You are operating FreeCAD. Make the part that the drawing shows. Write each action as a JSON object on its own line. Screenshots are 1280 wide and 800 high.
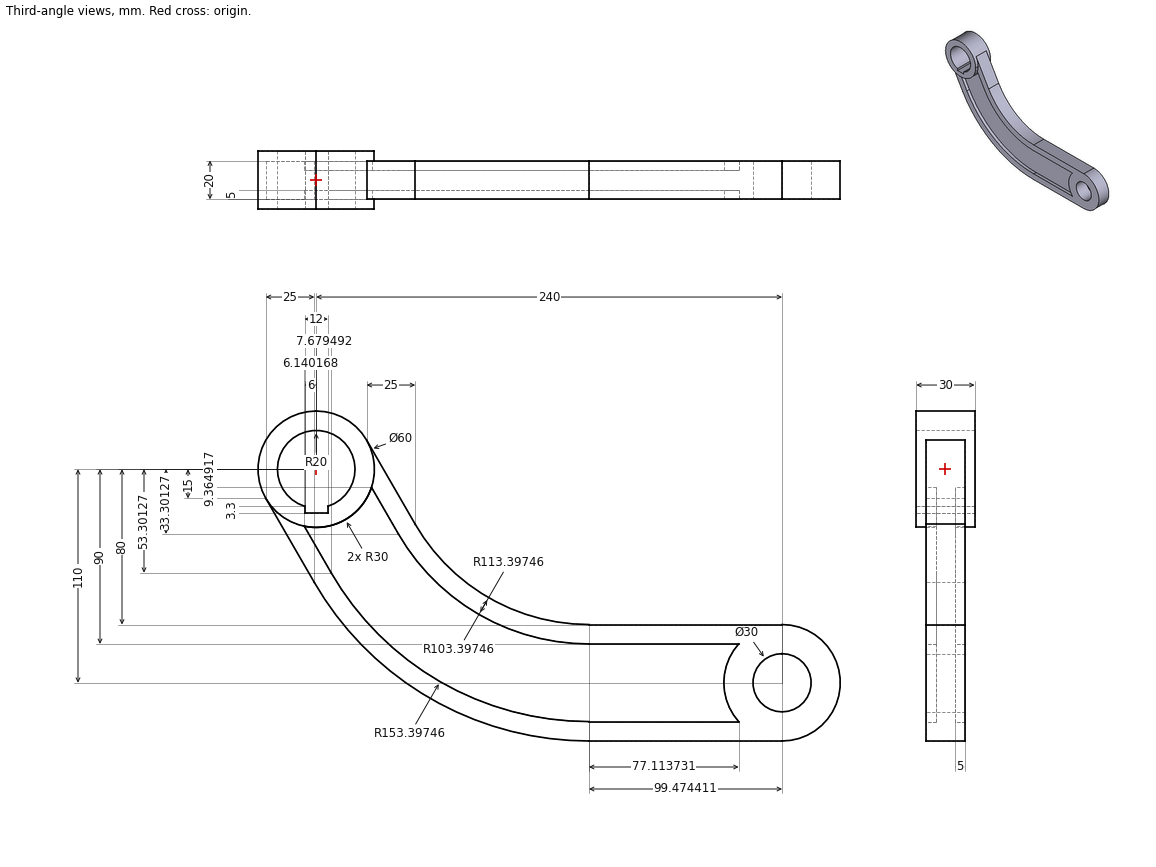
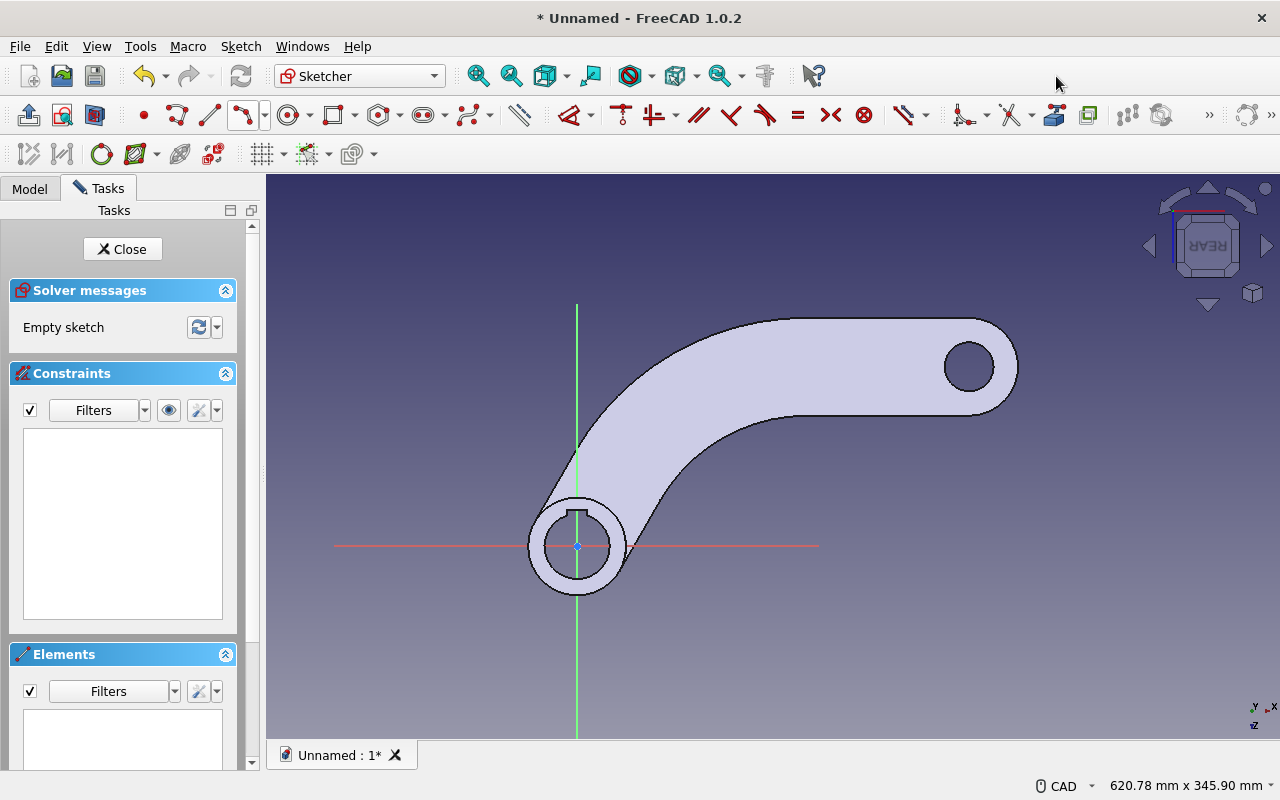
{"action": "scroll", "coordinate": [842, 407], "scroll_direction": "up", "scroll_amount": 2}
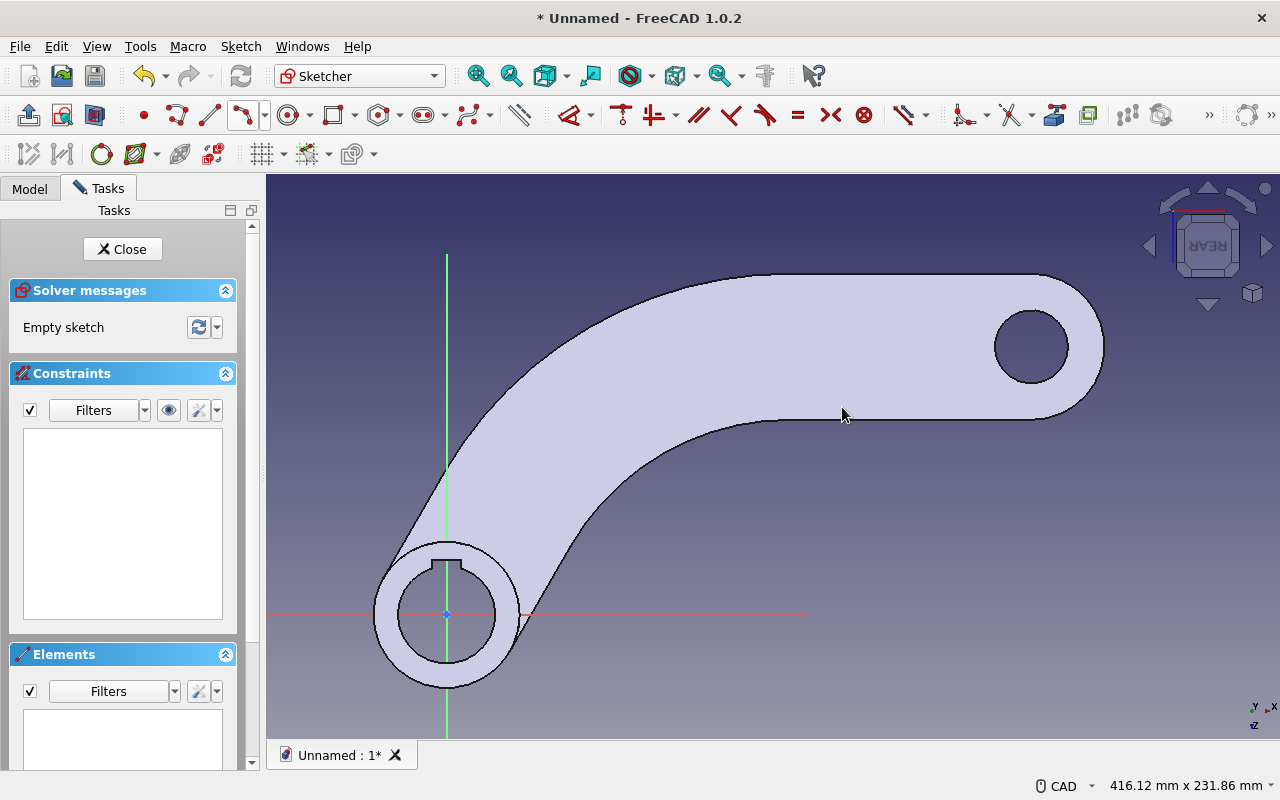
{"action": "left_click", "coordinate": [210, 116]}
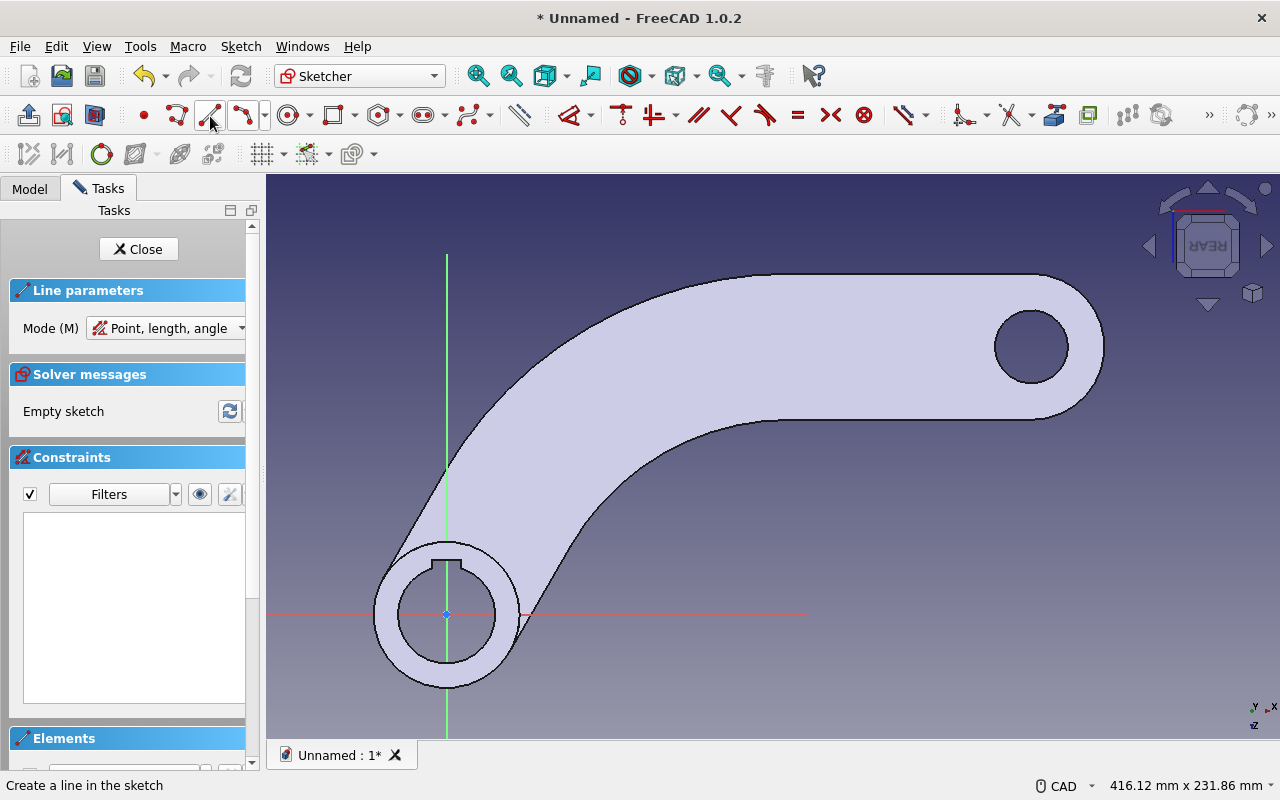
{"action": "left_click", "coordinate": [977, 298]}
{"action": "left_click", "coordinate": [789, 298]}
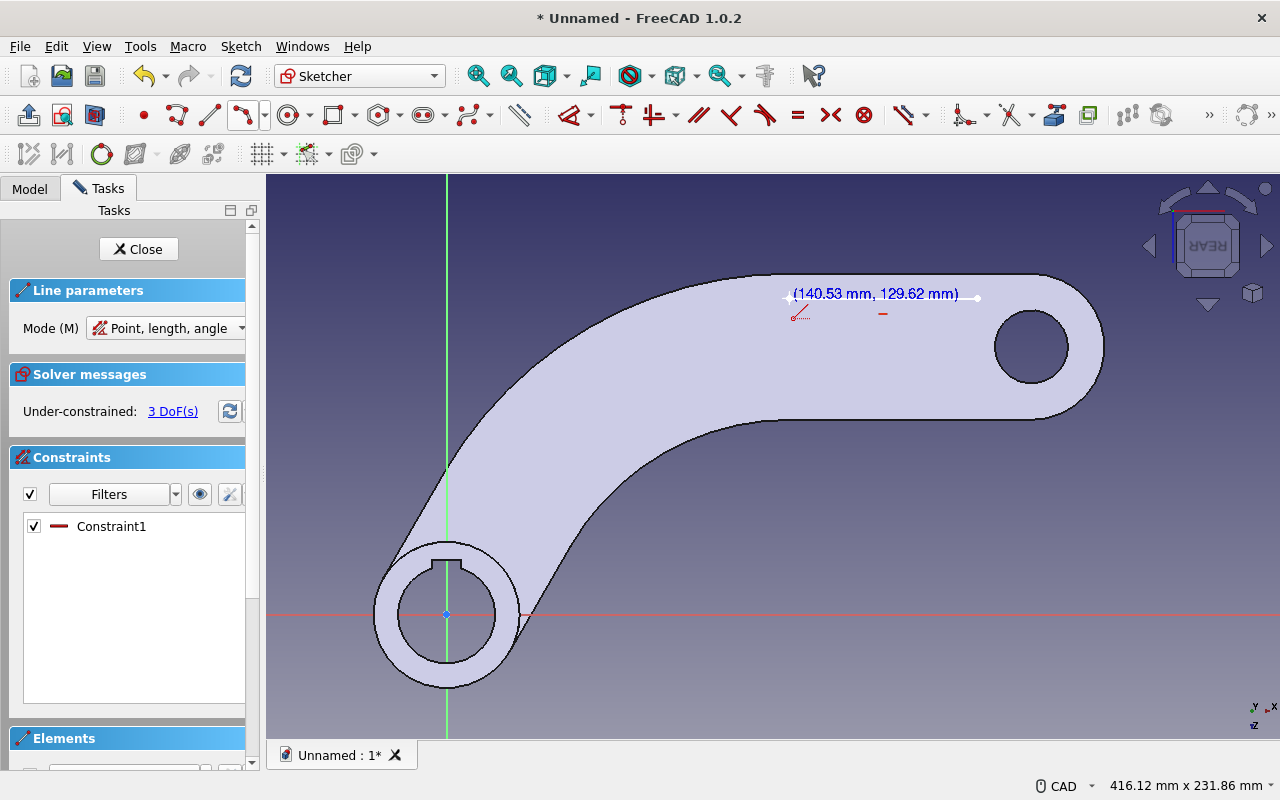
{"action": "left_click", "coordinate": [465, 485]}
{"action": "left_click", "coordinate": [432, 543]}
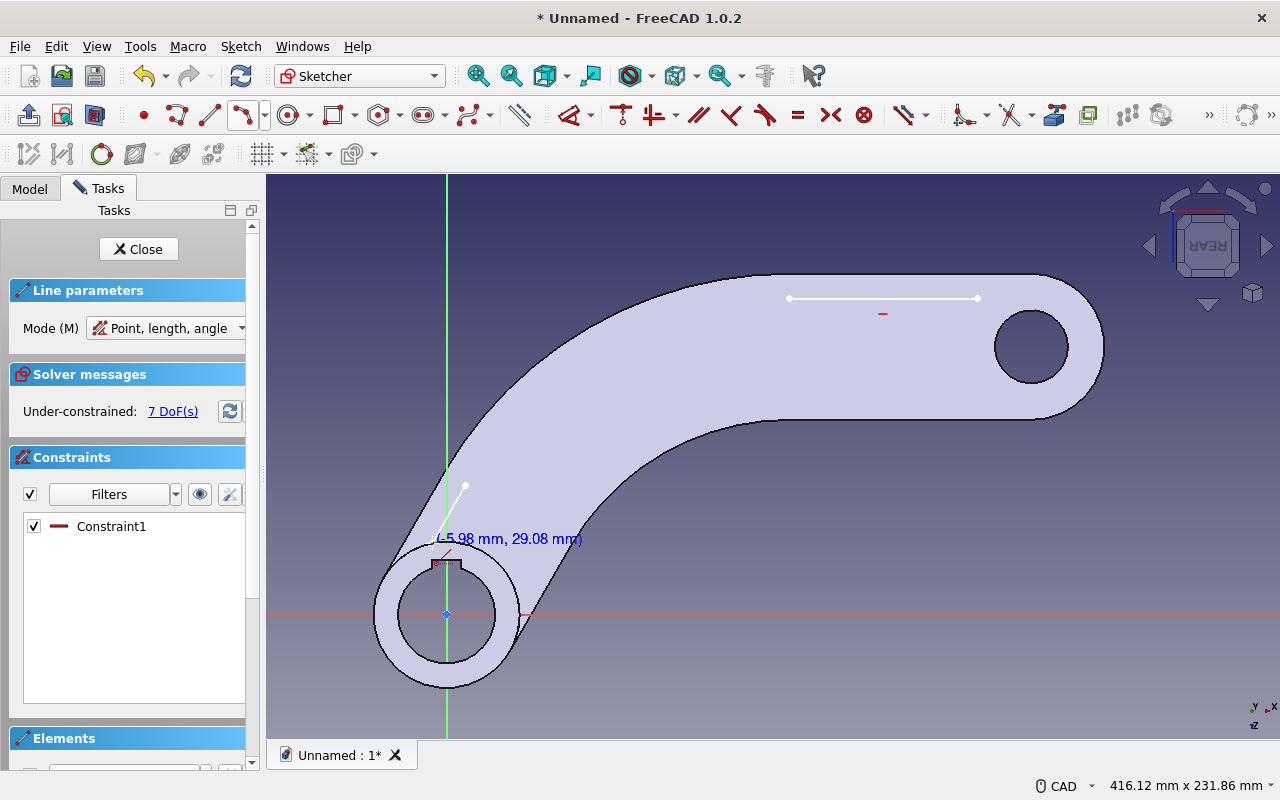
{"action": "left_click", "coordinate": [516, 592]}
{"action": "left_click", "coordinate": [550, 534]}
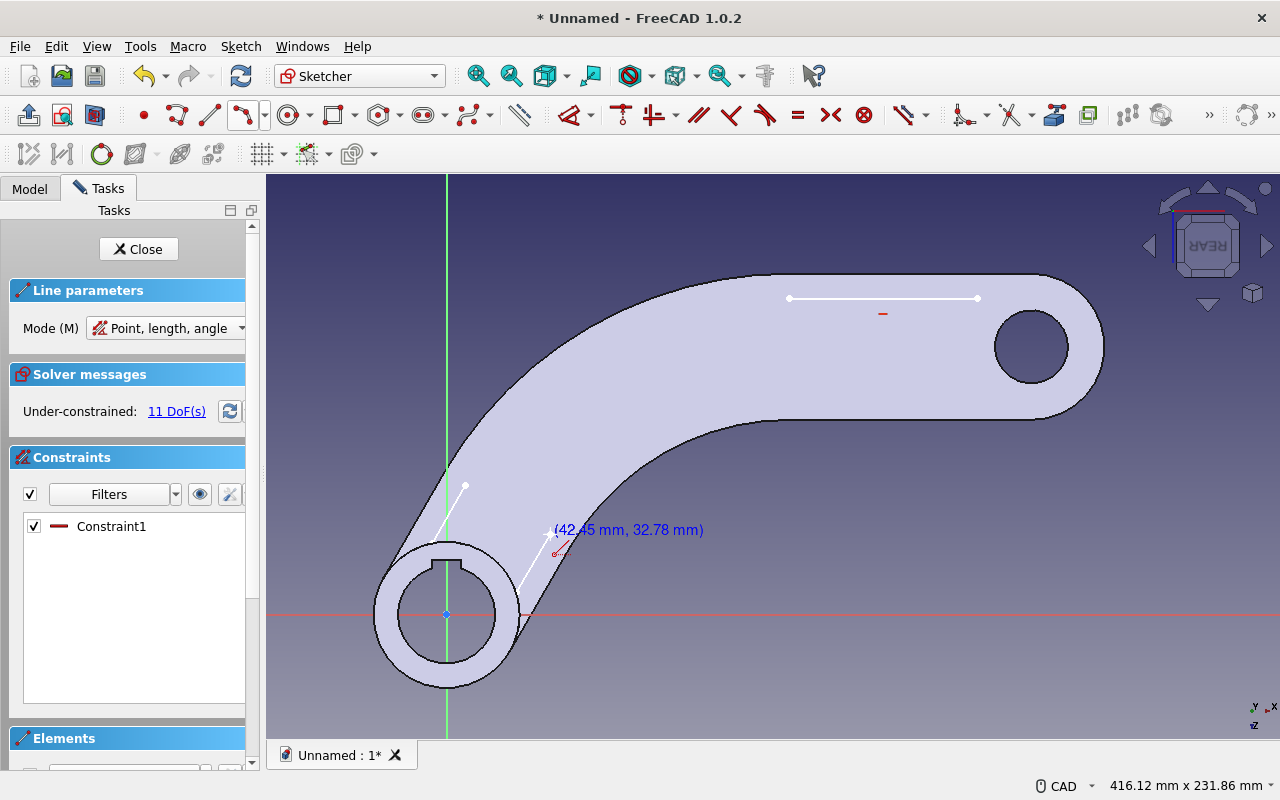
{"action": "left_click", "coordinate": [789, 396]}
{"action": "left_click", "coordinate": [977, 396]}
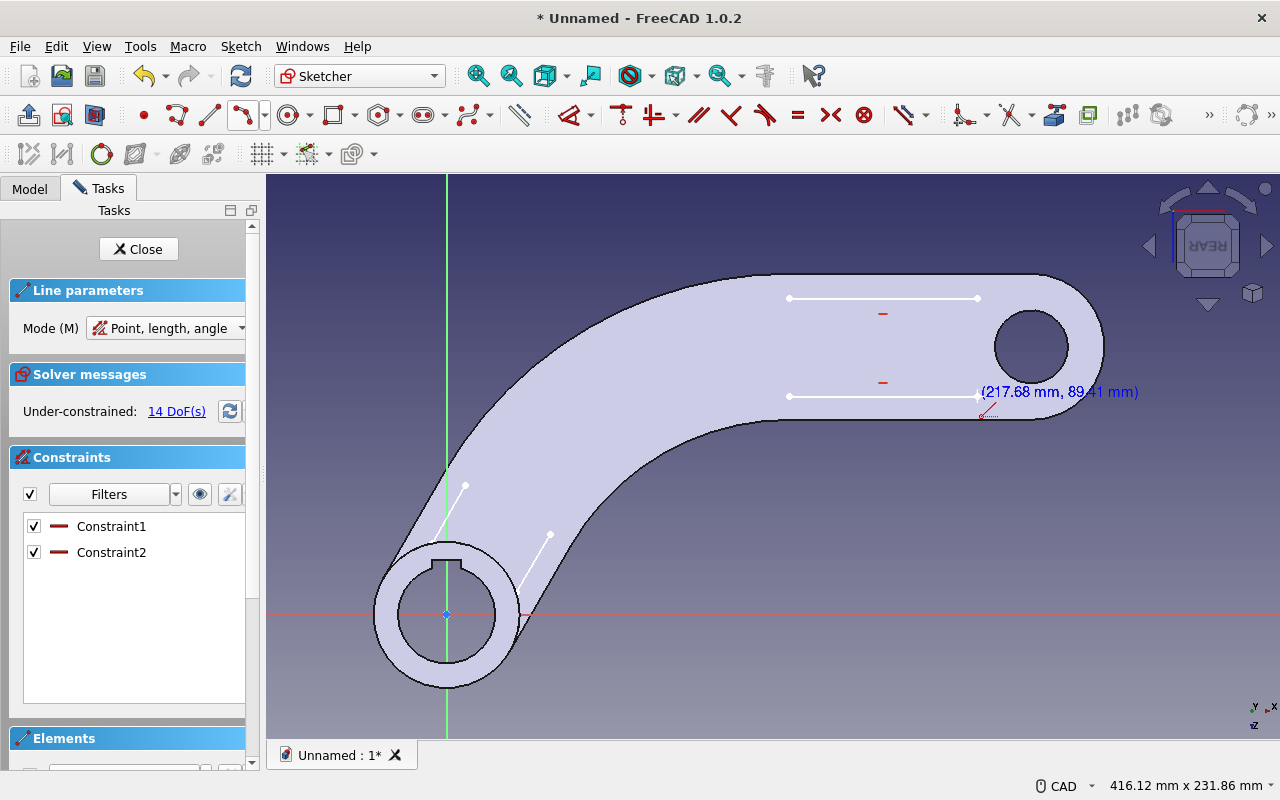
{"action": "left_click", "coordinate": [242, 116]}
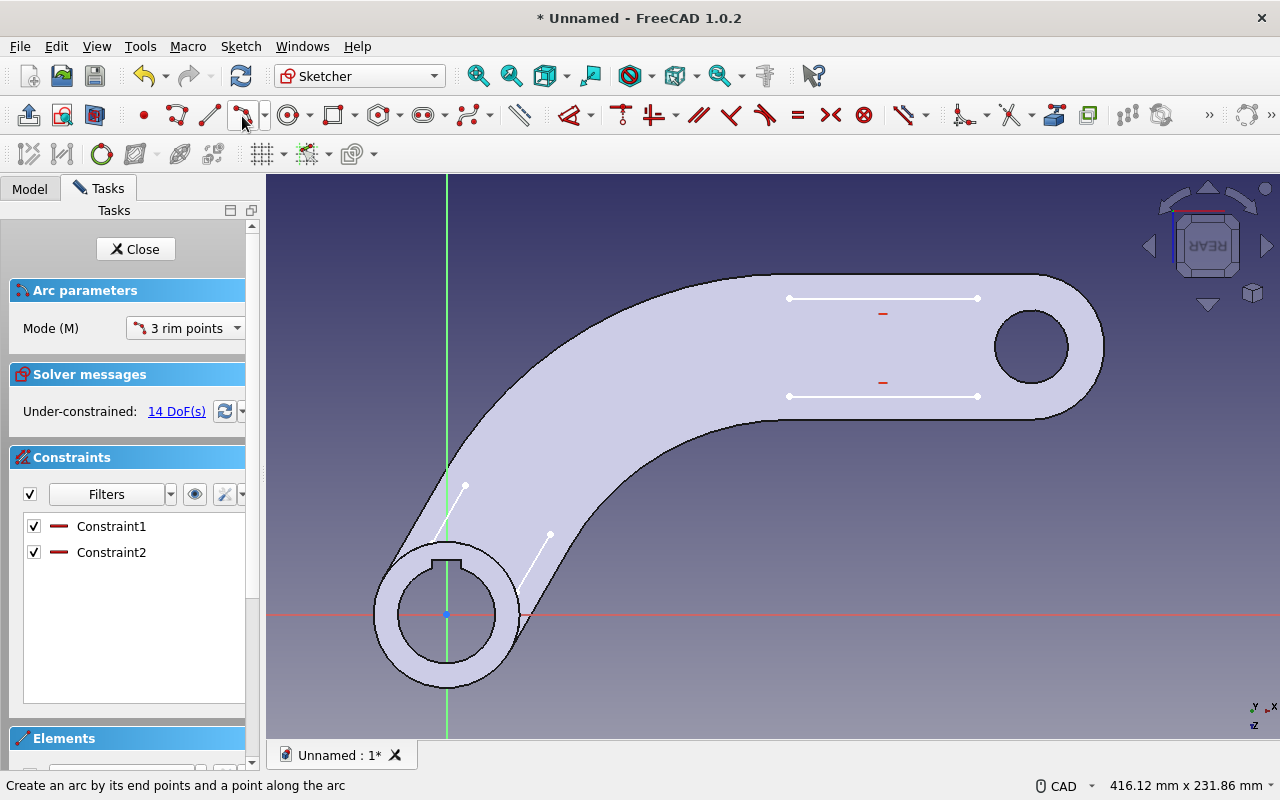
{"action": "left_click", "coordinate": [789, 299]}
{"action": "left_click", "coordinate": [465, 486]}
{"action": "left_click", "coordinate": [602, 348]}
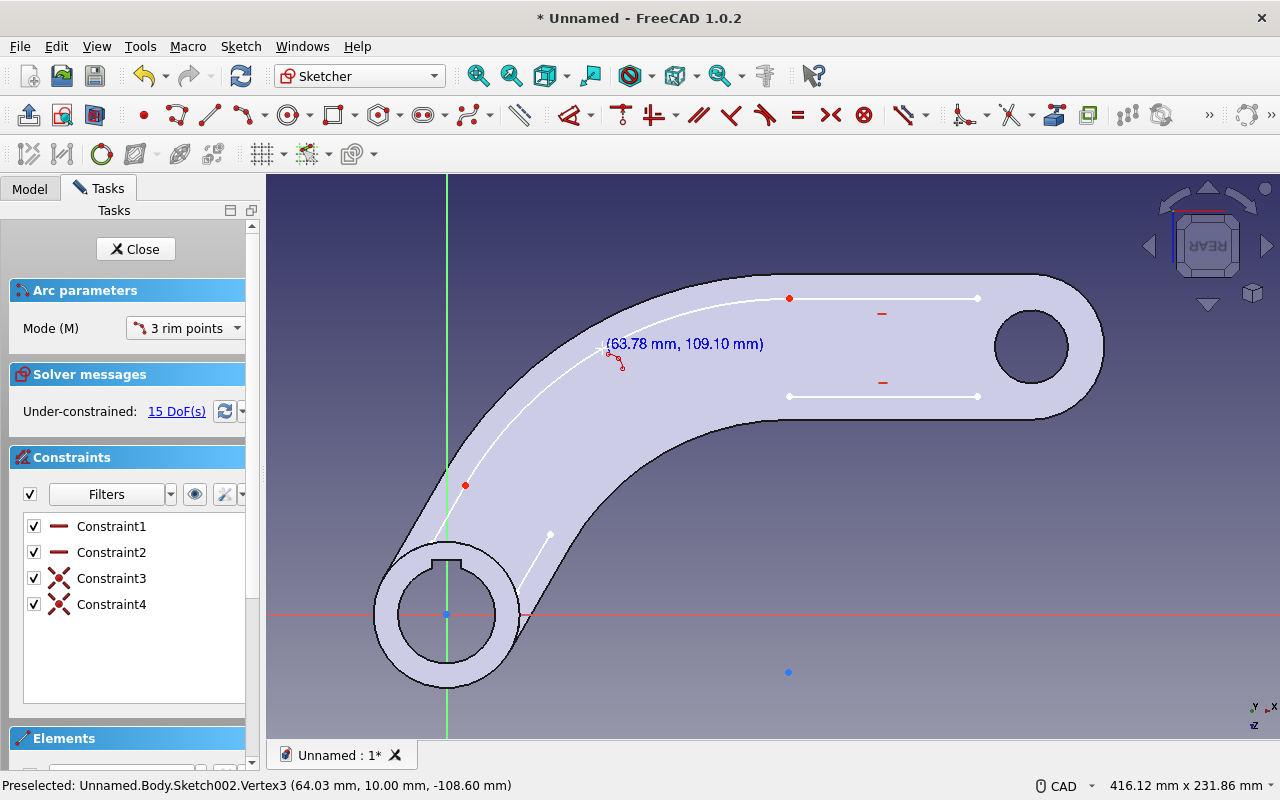
{"action": "left_click", "coordinate": [432, 544]}
{"action": "left_click", "coordinate": [516, 593]}
{"action": "left_click", "coordinate": [483, 552]}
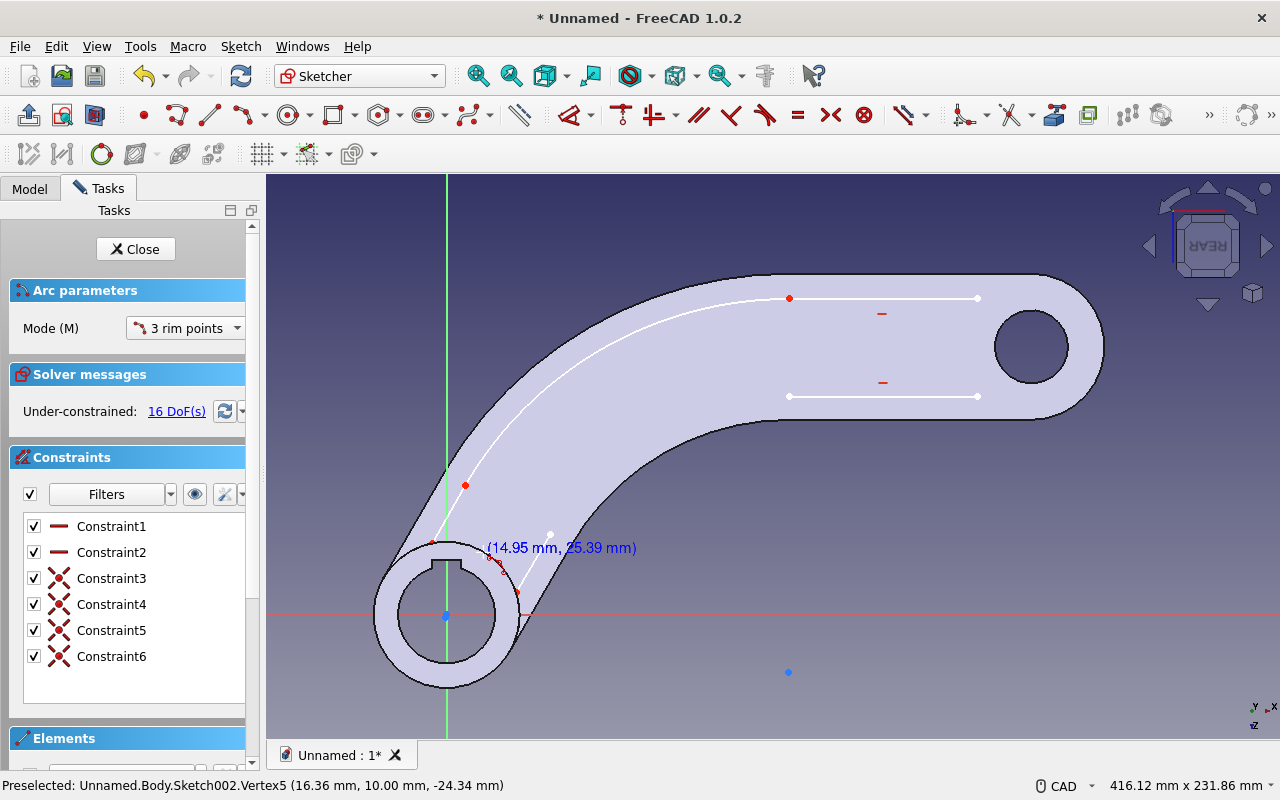
{"action": "left_click", "coordinate": [550, 535]}
{"action": "left_click", "coordinate": [789, 397]}
{"action": "left_click", "coordinate": [651, 433]}